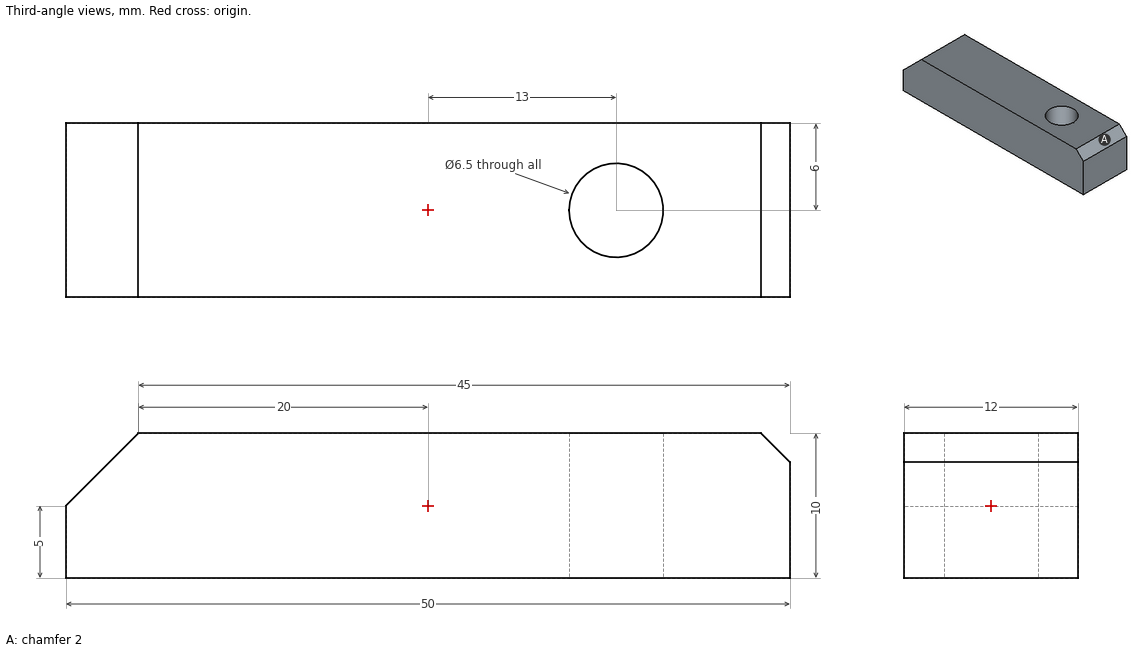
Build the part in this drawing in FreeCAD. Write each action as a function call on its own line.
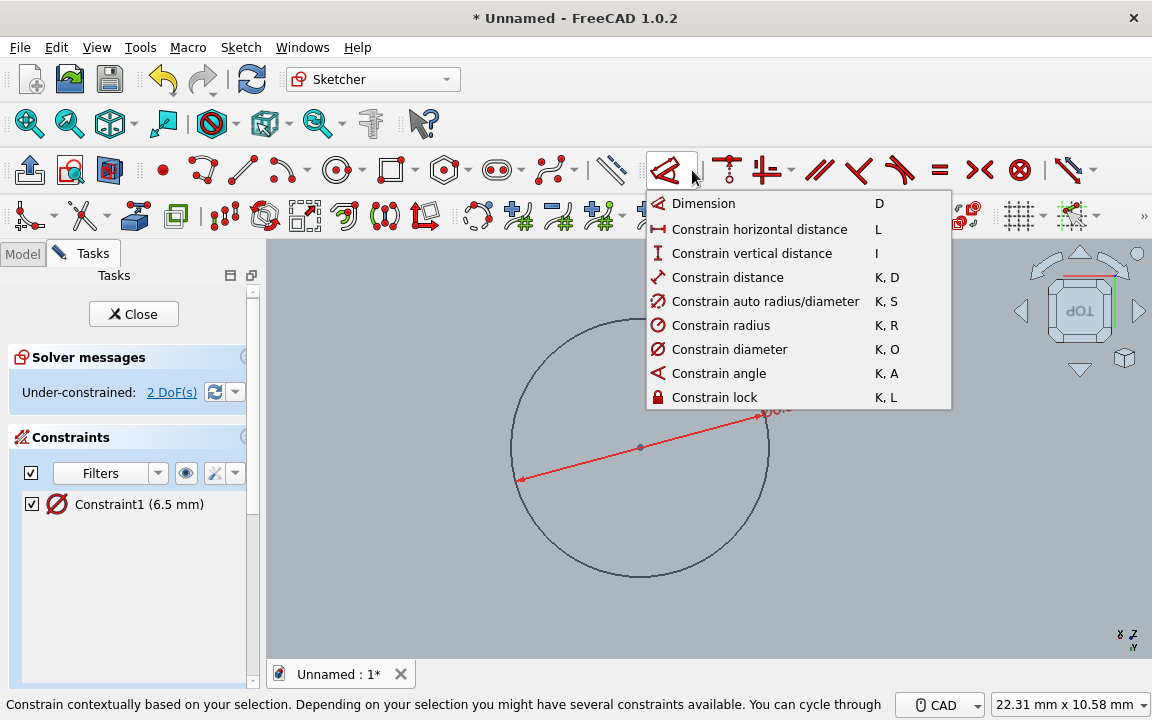
click(799, 253)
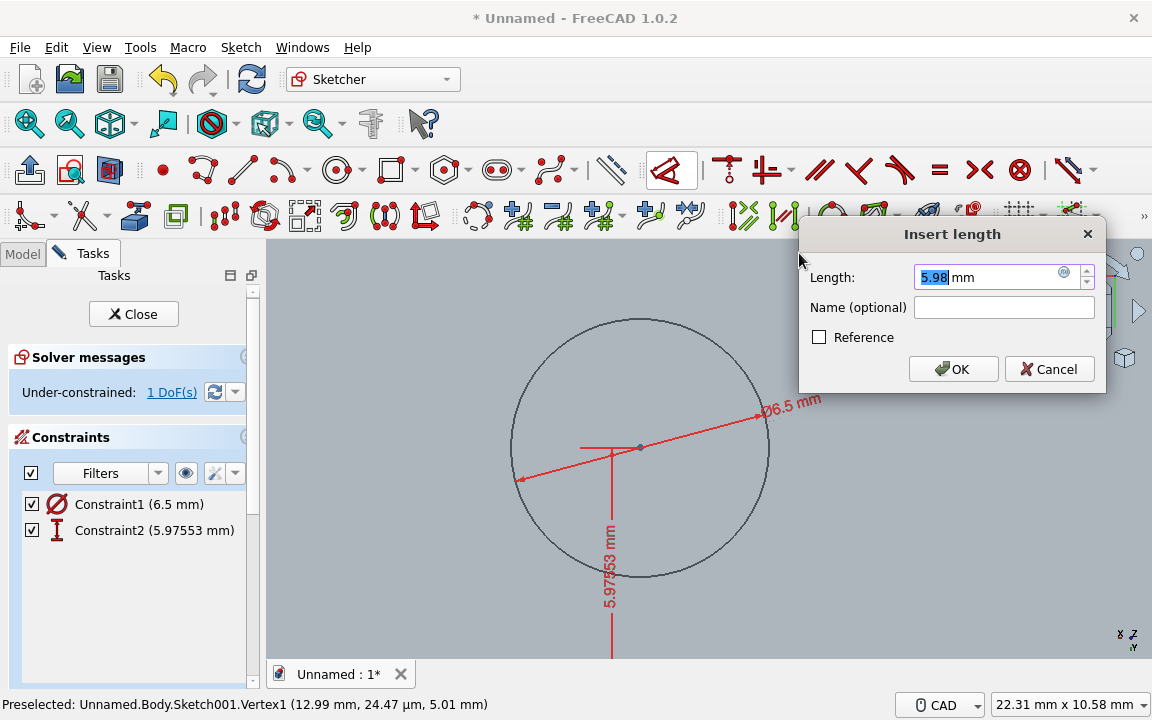
text(6)
key(Return)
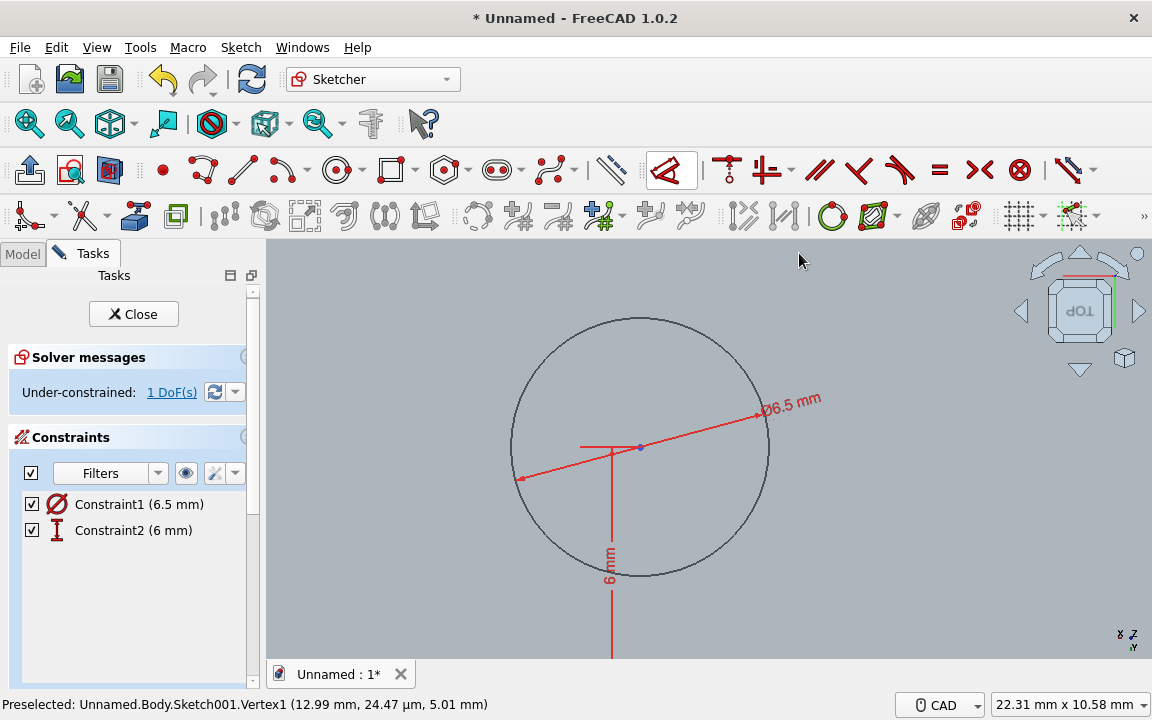
click(640, 447)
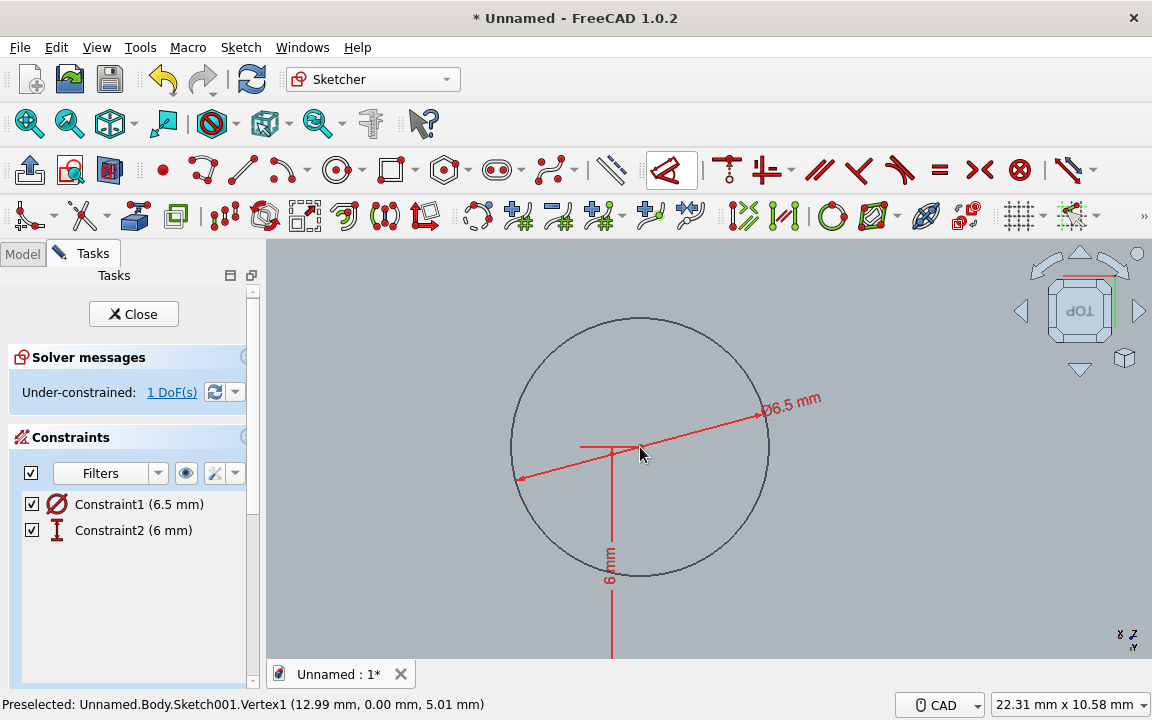
click(692, 170)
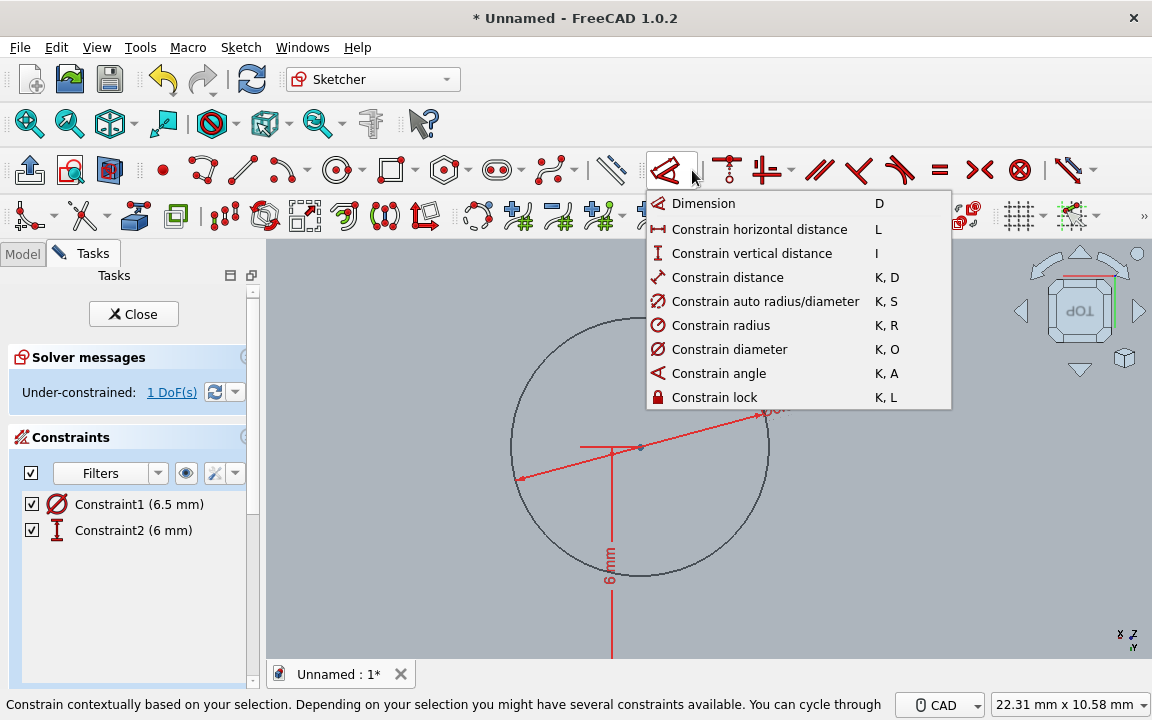
click(799, 229)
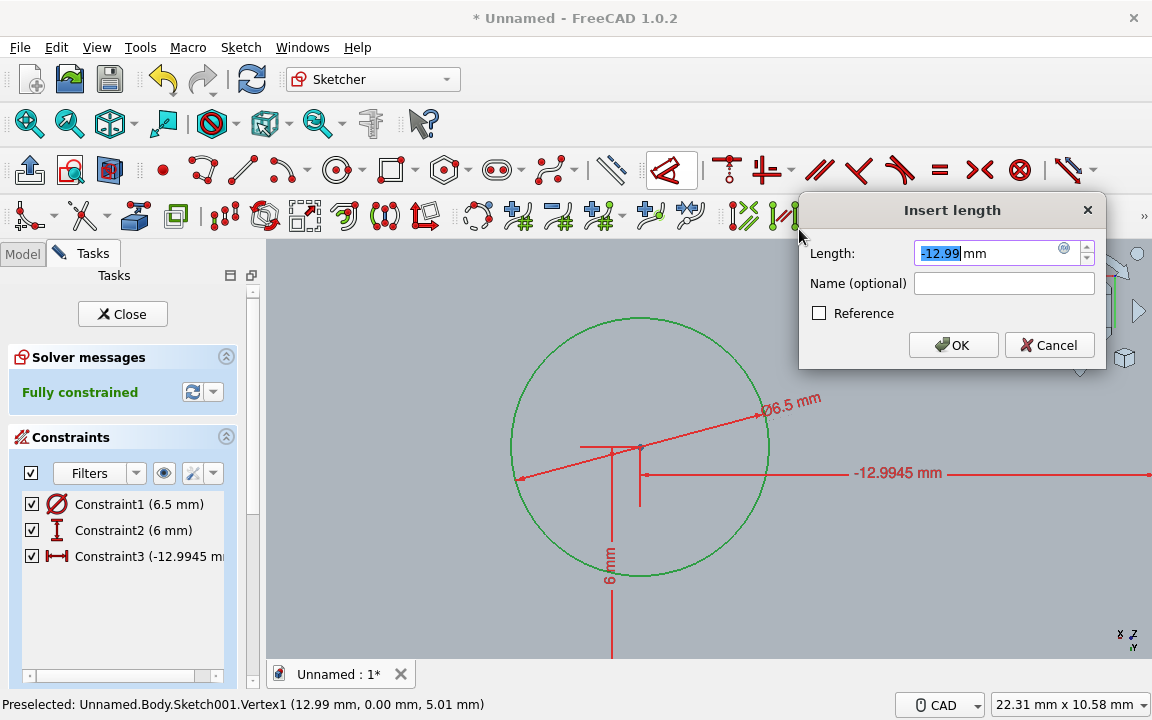
text(-13)
key(Return)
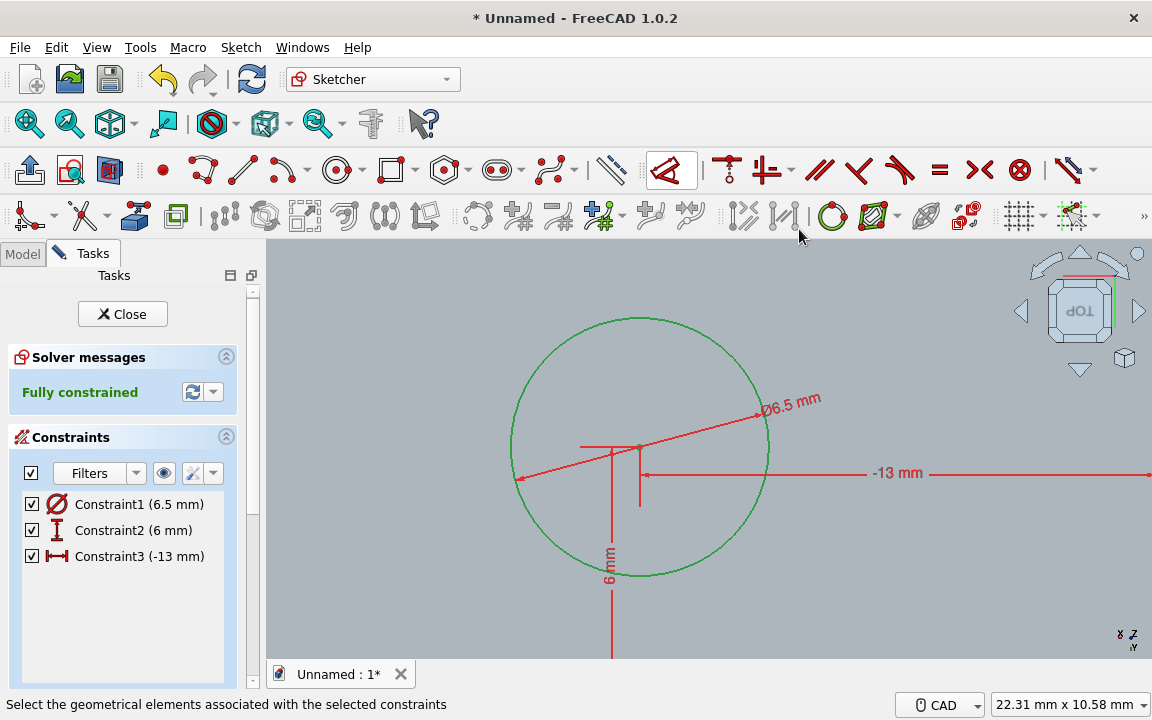
click(123, 314)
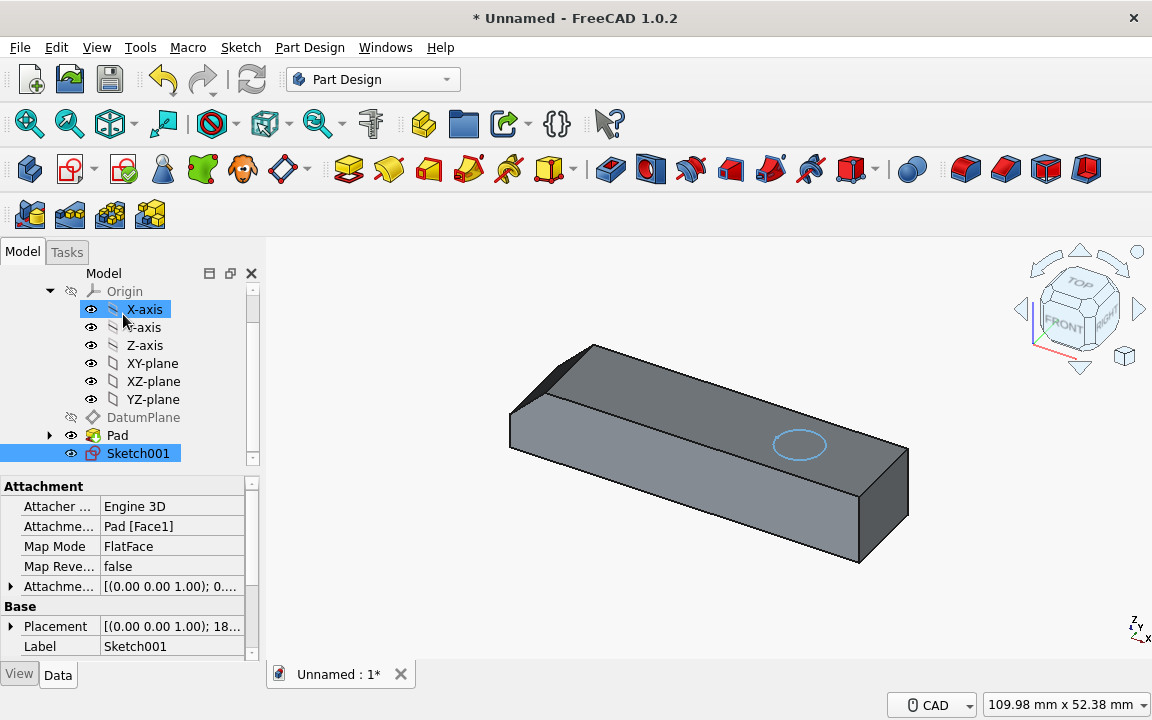
click(652, 170)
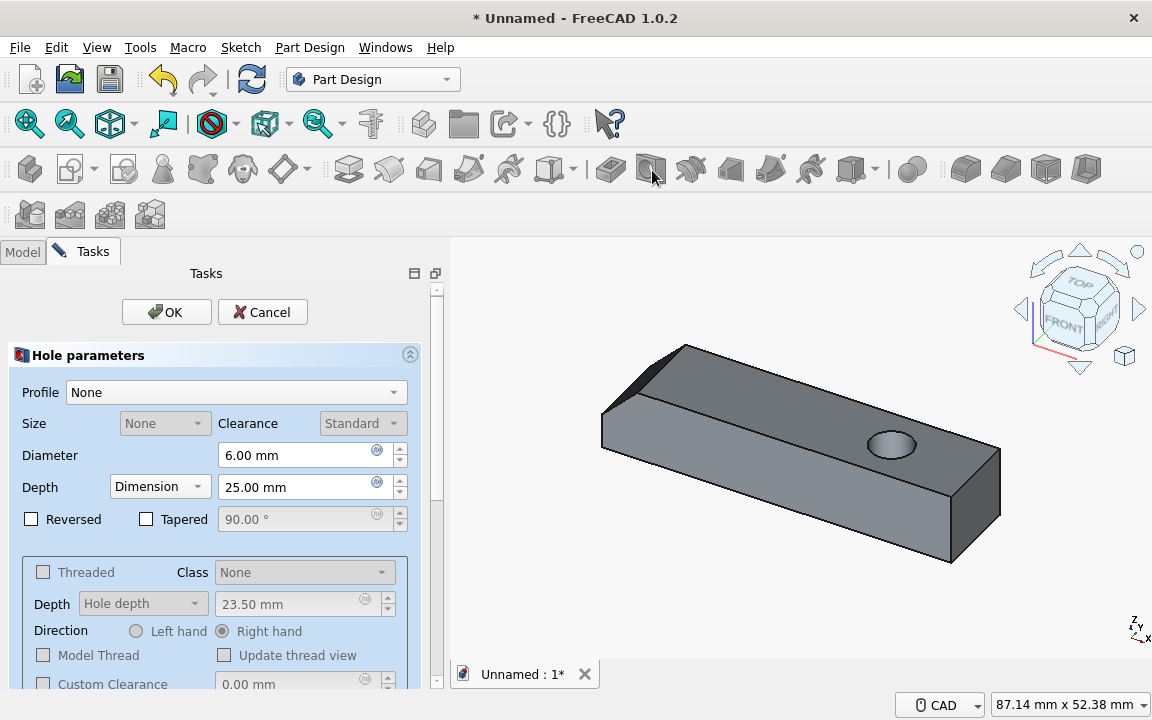
triple_click(305, 455)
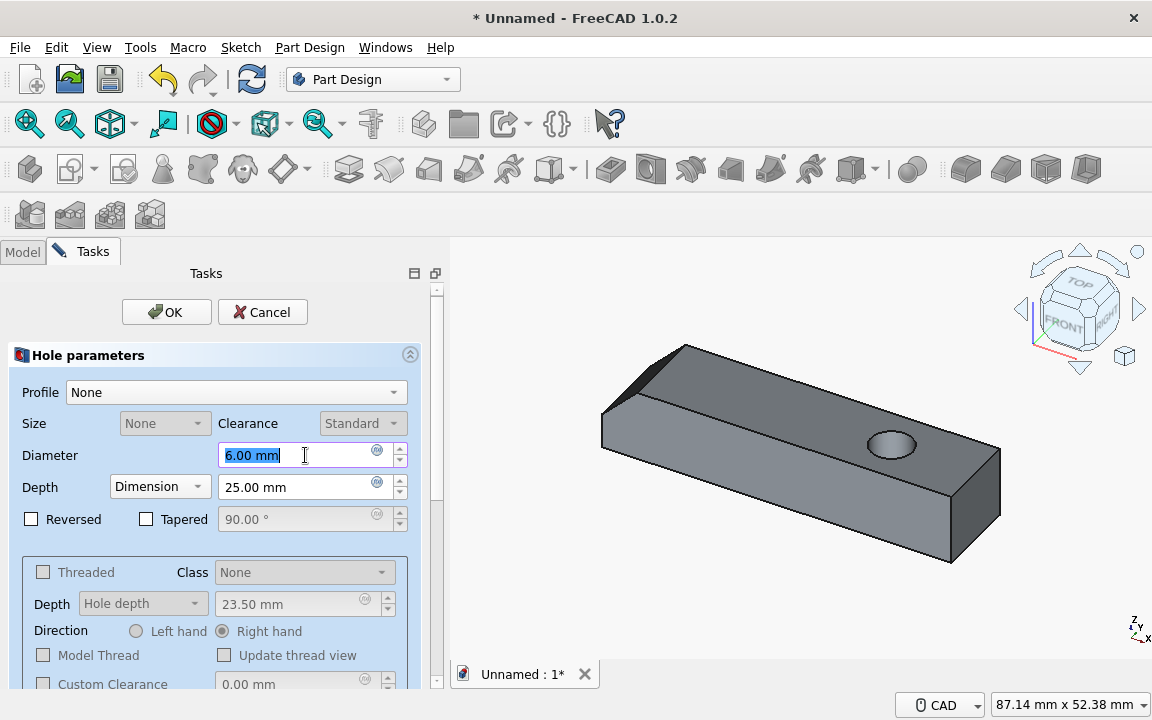
text(6.5)
key(Tab)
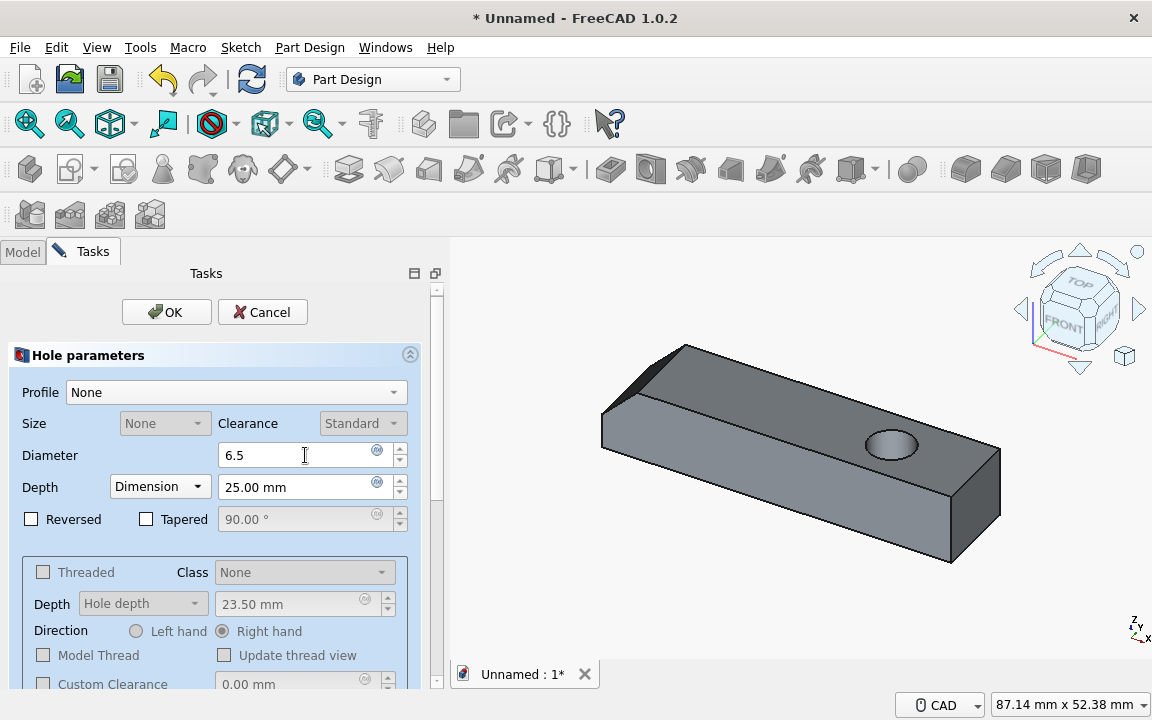
click(161, 486)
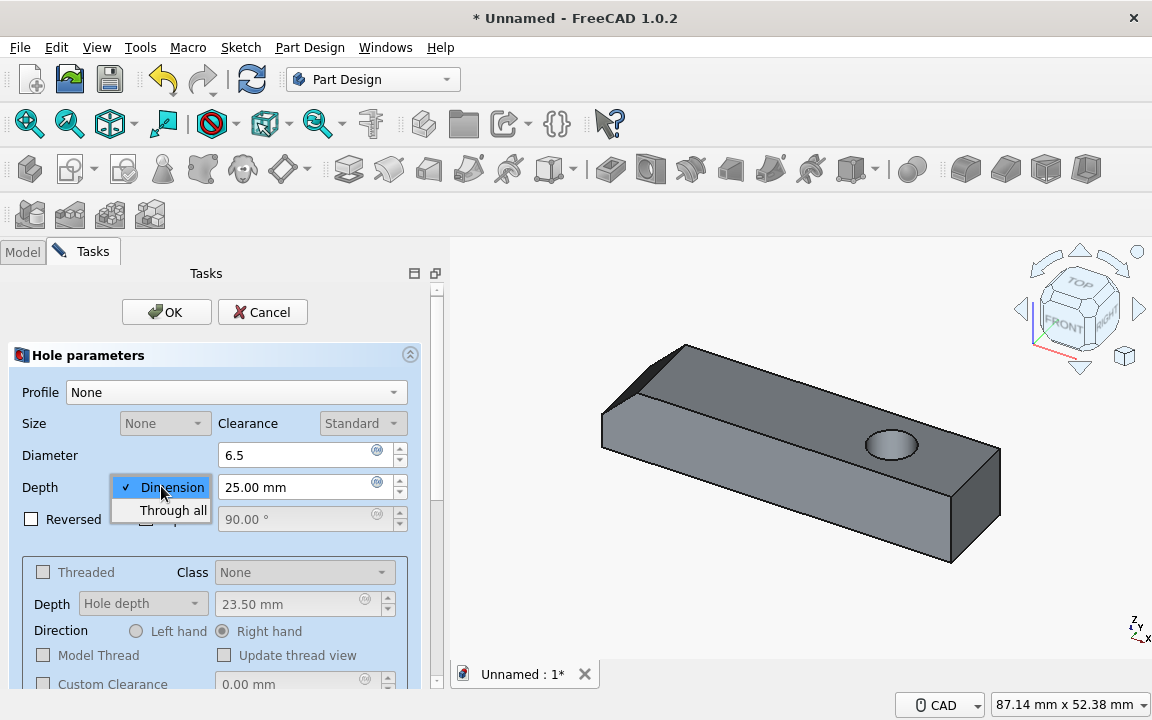
click(160, 510)